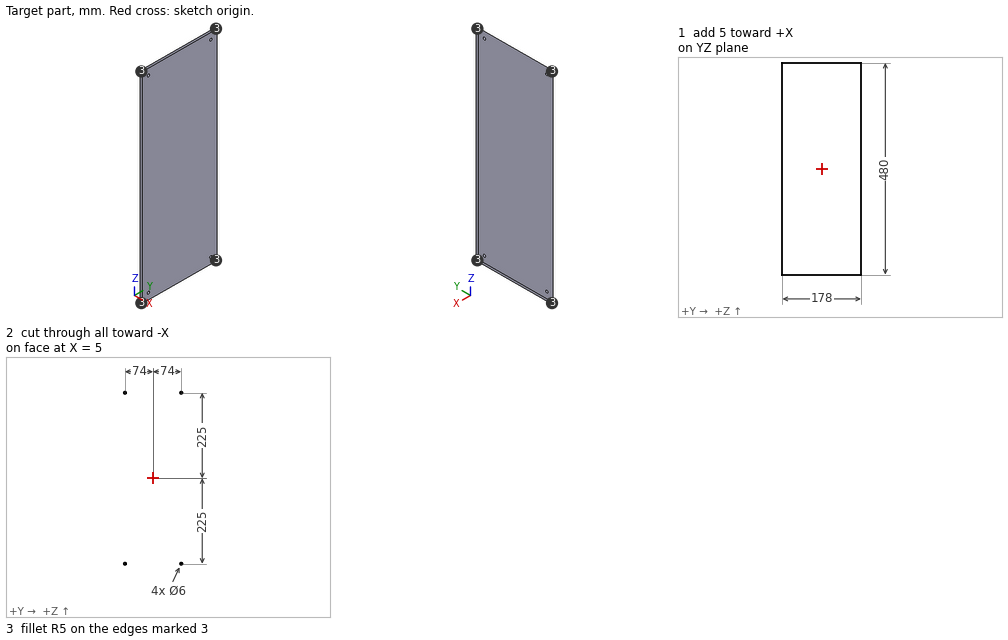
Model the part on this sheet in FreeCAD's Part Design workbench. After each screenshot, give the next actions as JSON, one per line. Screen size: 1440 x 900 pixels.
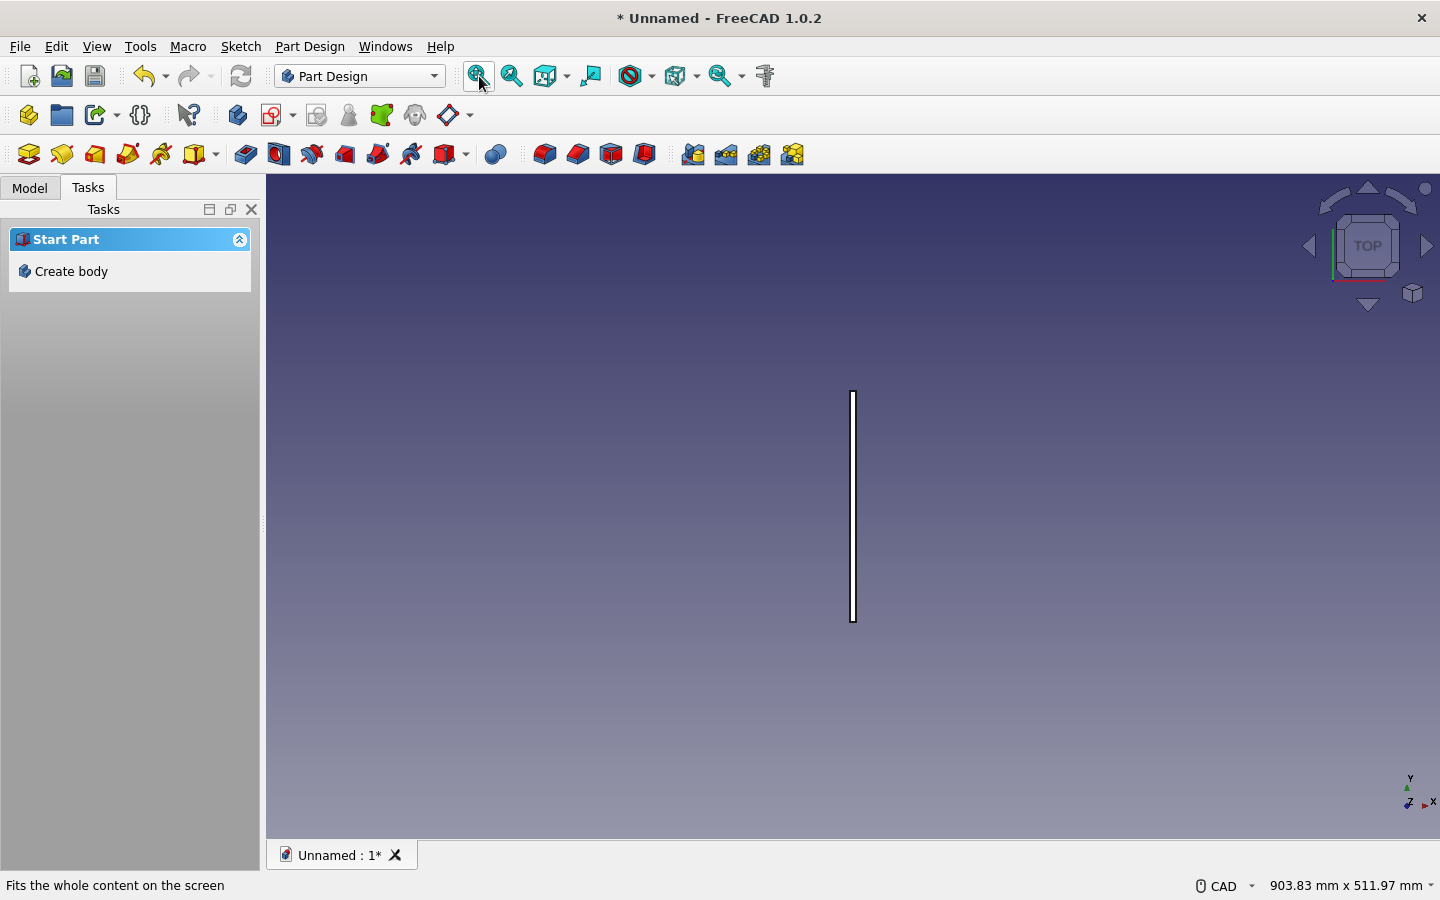
{"action": "left_click", "coordinate": [479, 76]}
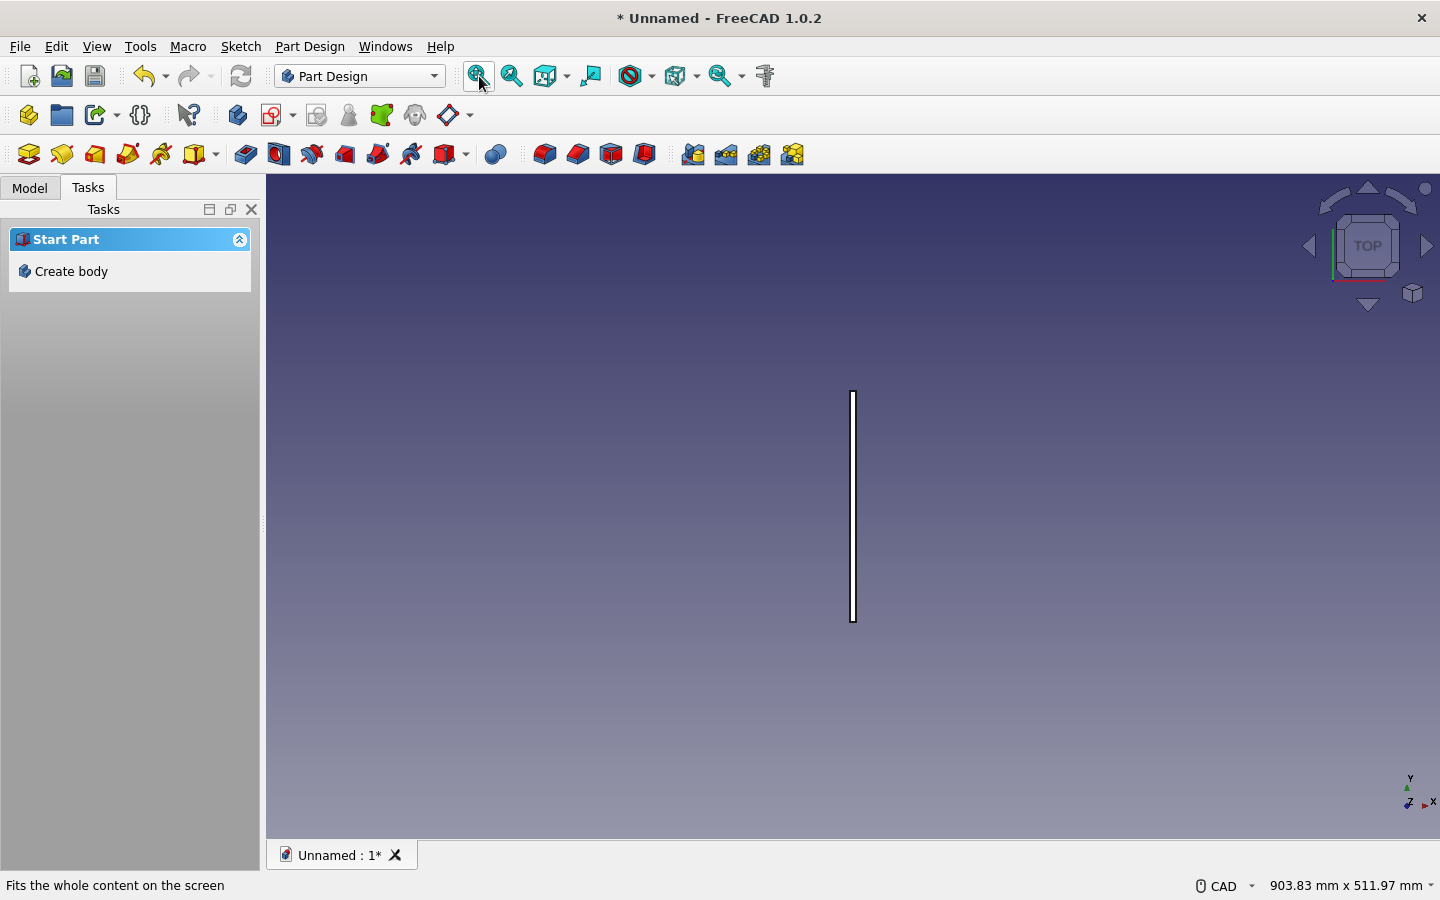
{"action": "scroll", "coordinate": [853, 390], "scroll_direction": "up", "scroll_amount": 10}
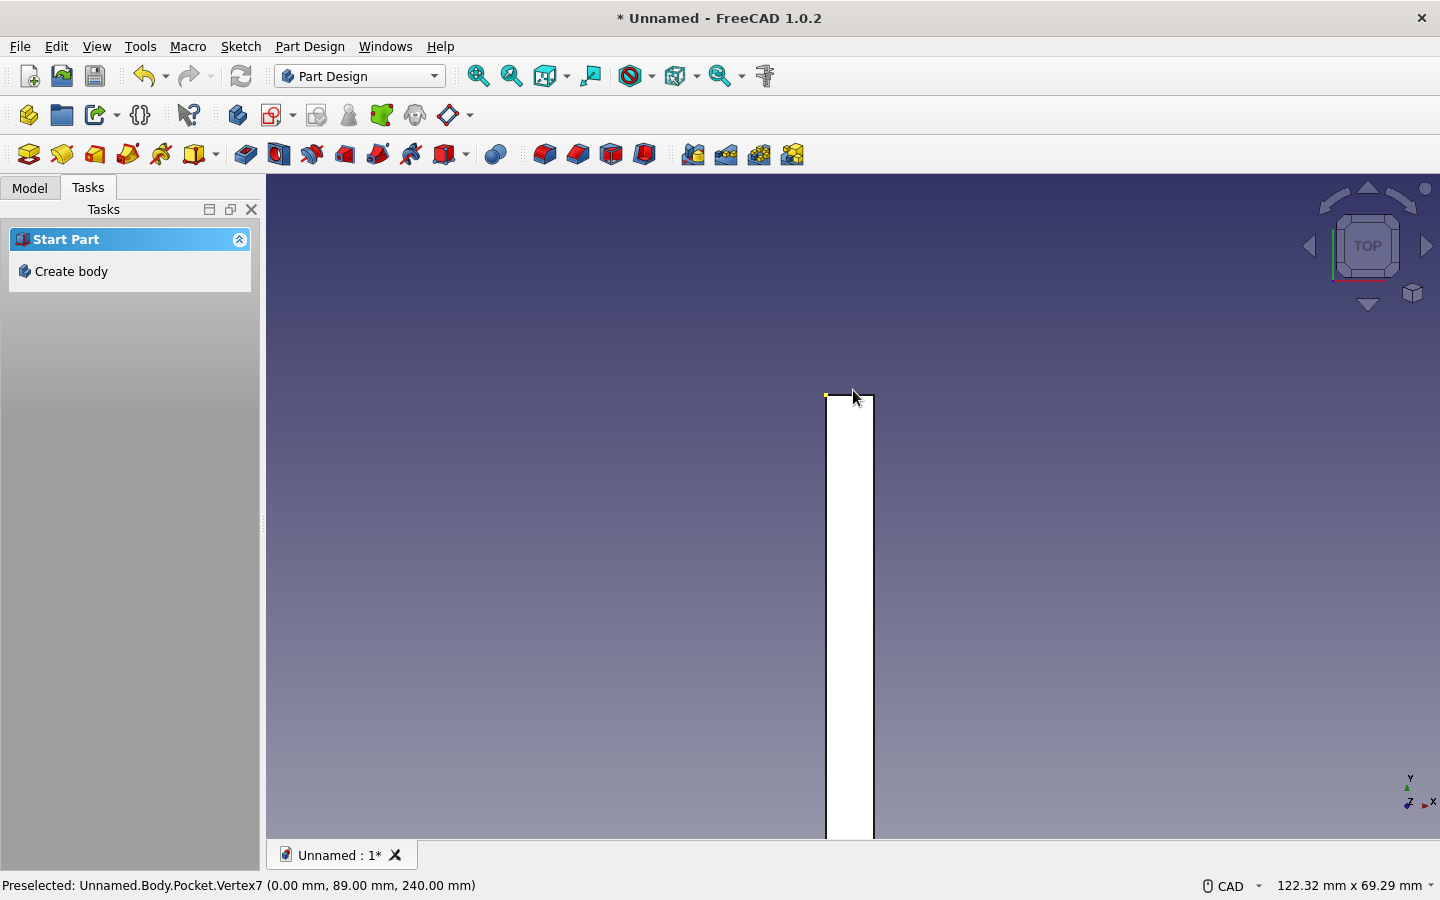
{"action": "left_click", "coordinate": [850, 394]}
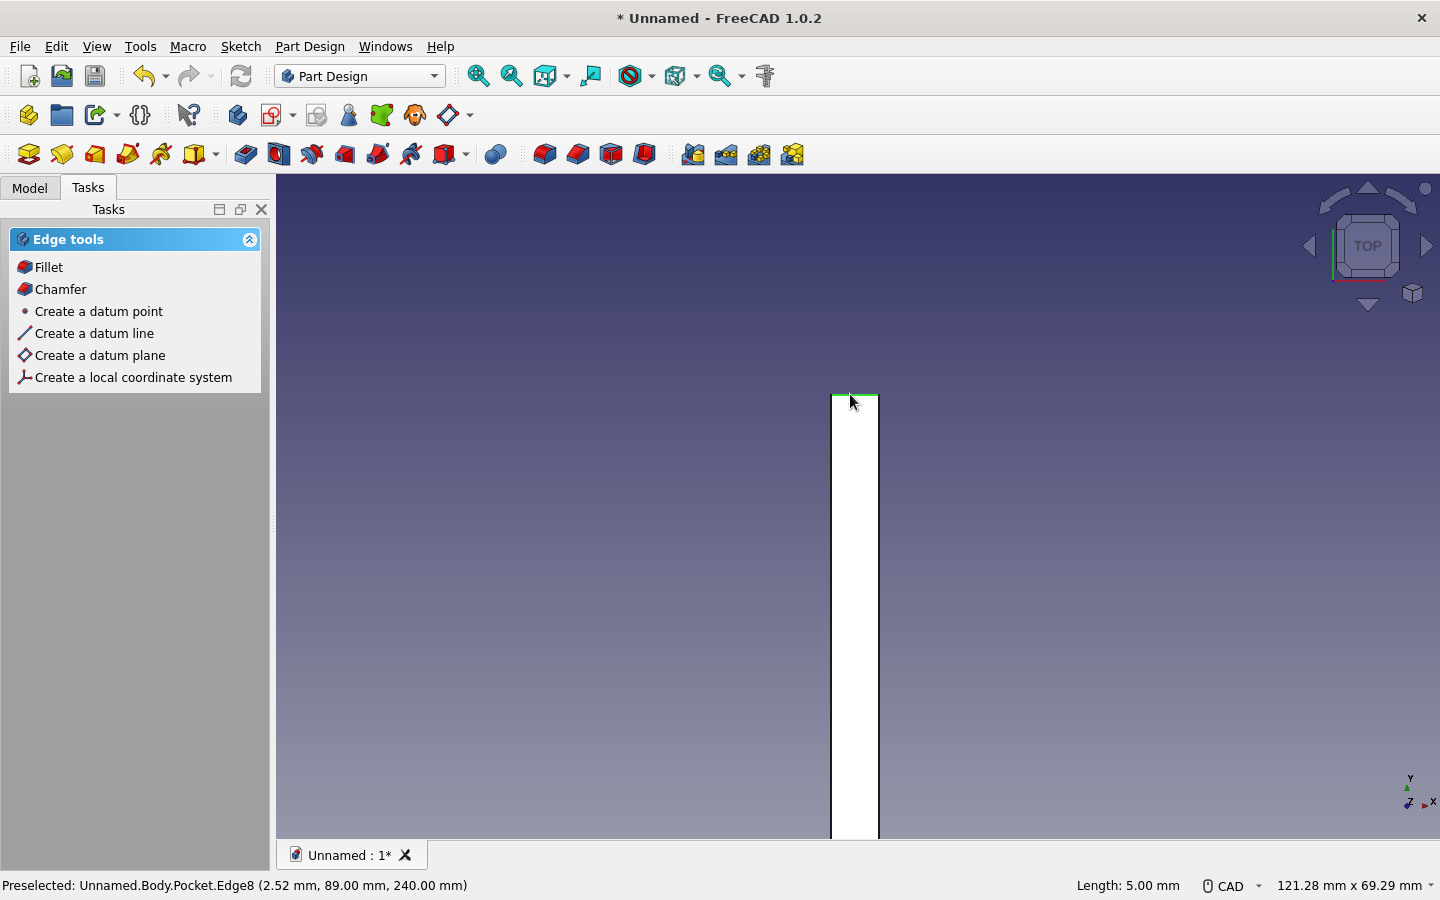
{"action": "left_click", "coordinate": [479, 76]}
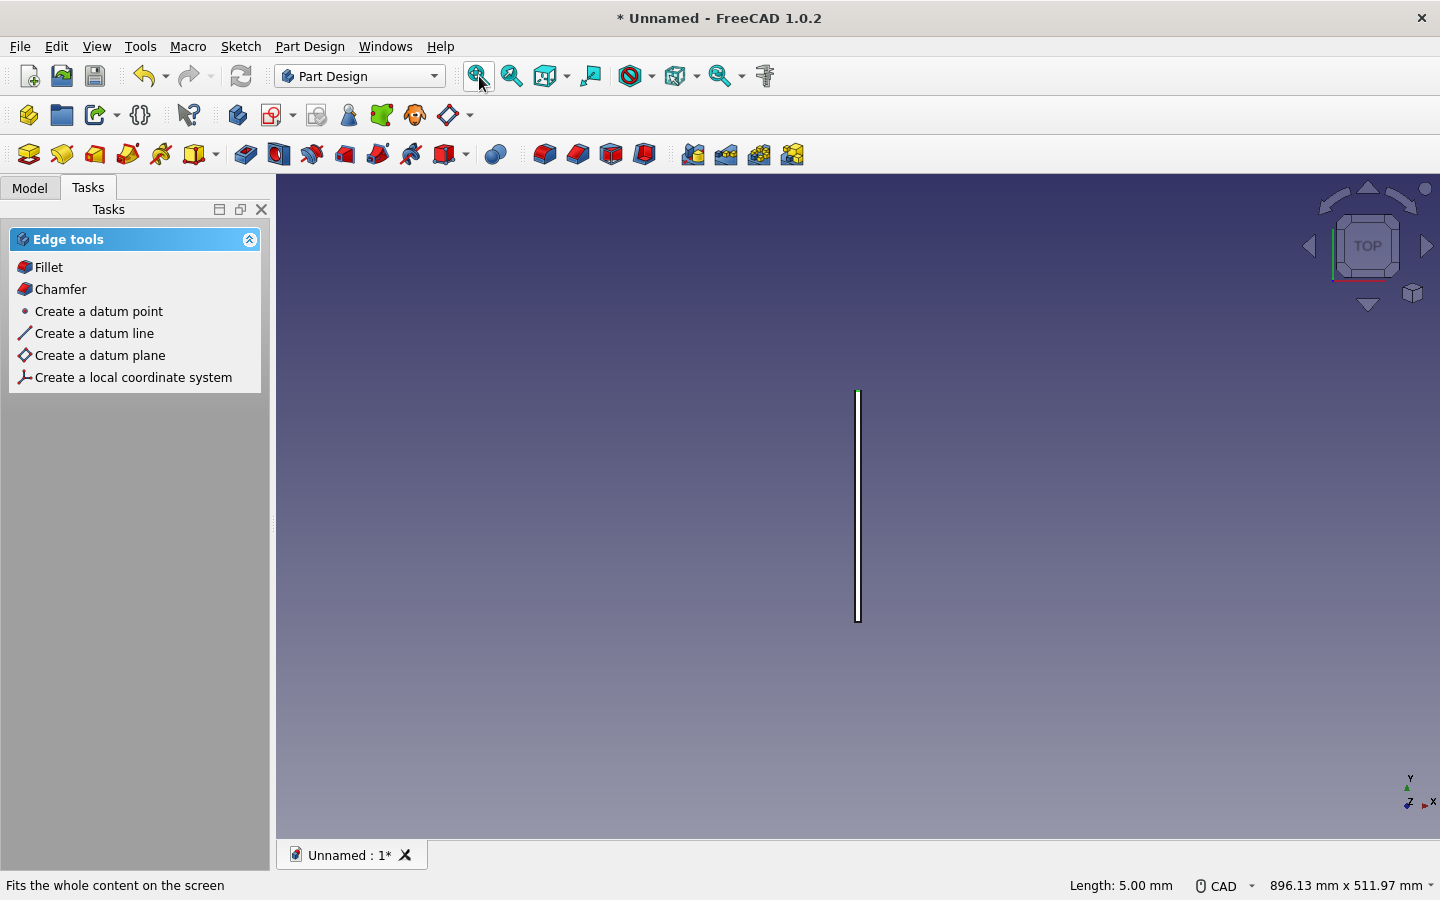
{"action": "key", "text": "1"}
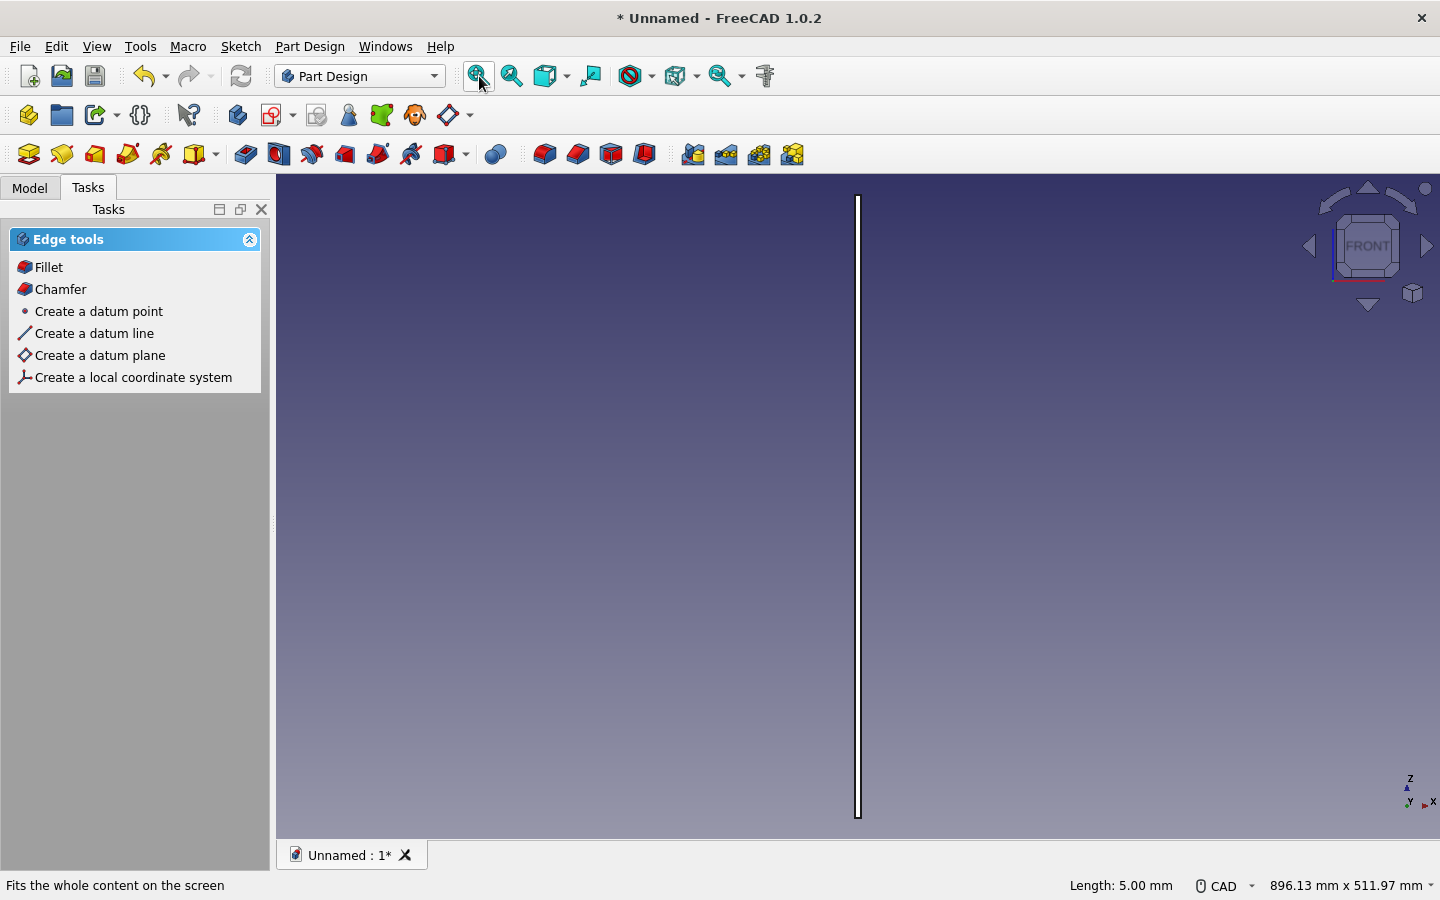
{"action": "key", "text": "3"}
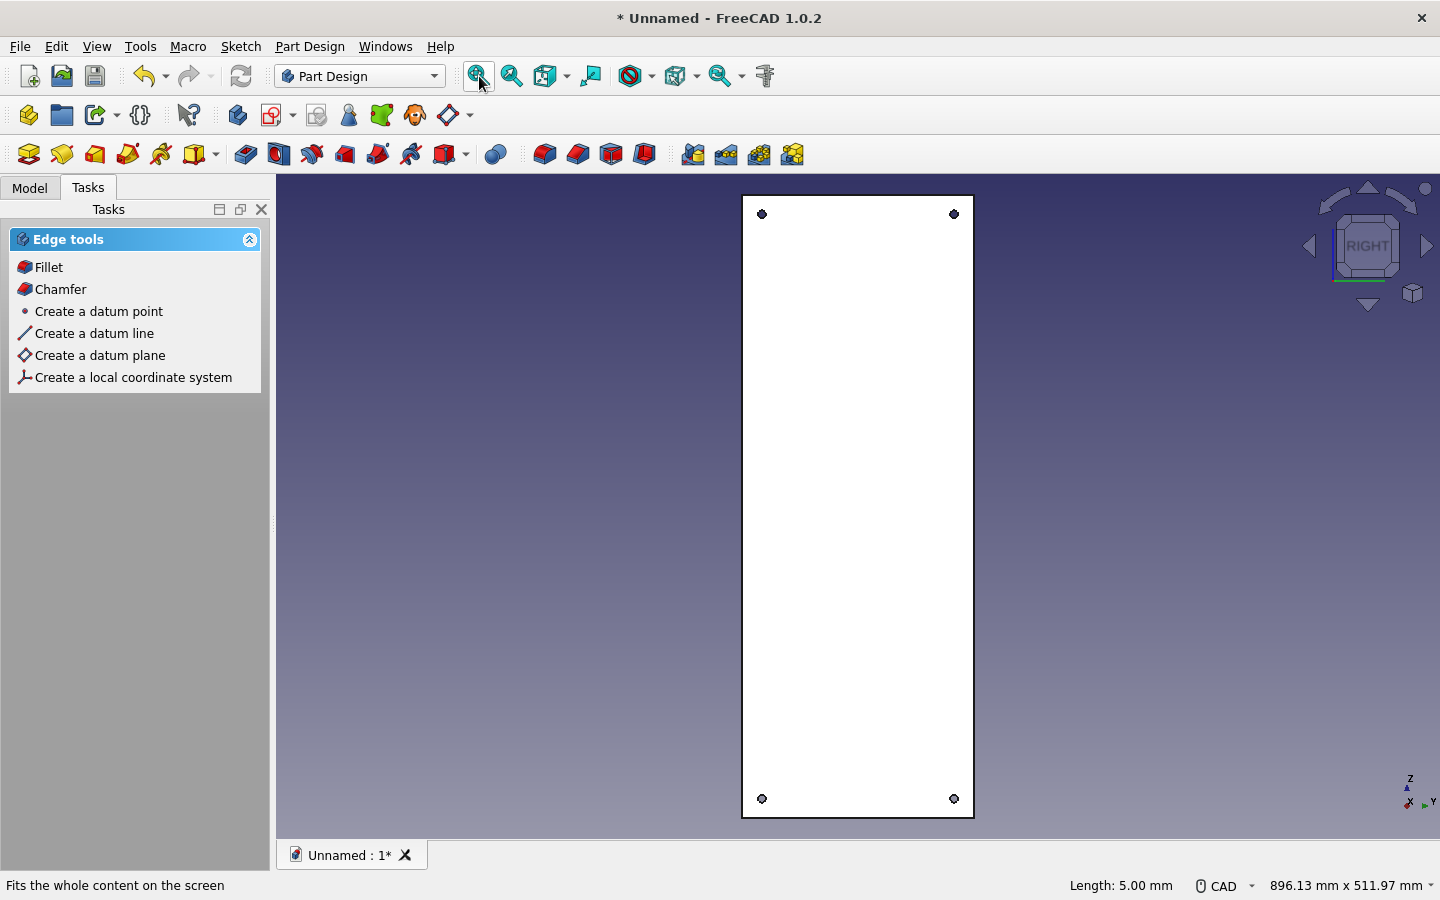
{"action": "key", "text": "5"}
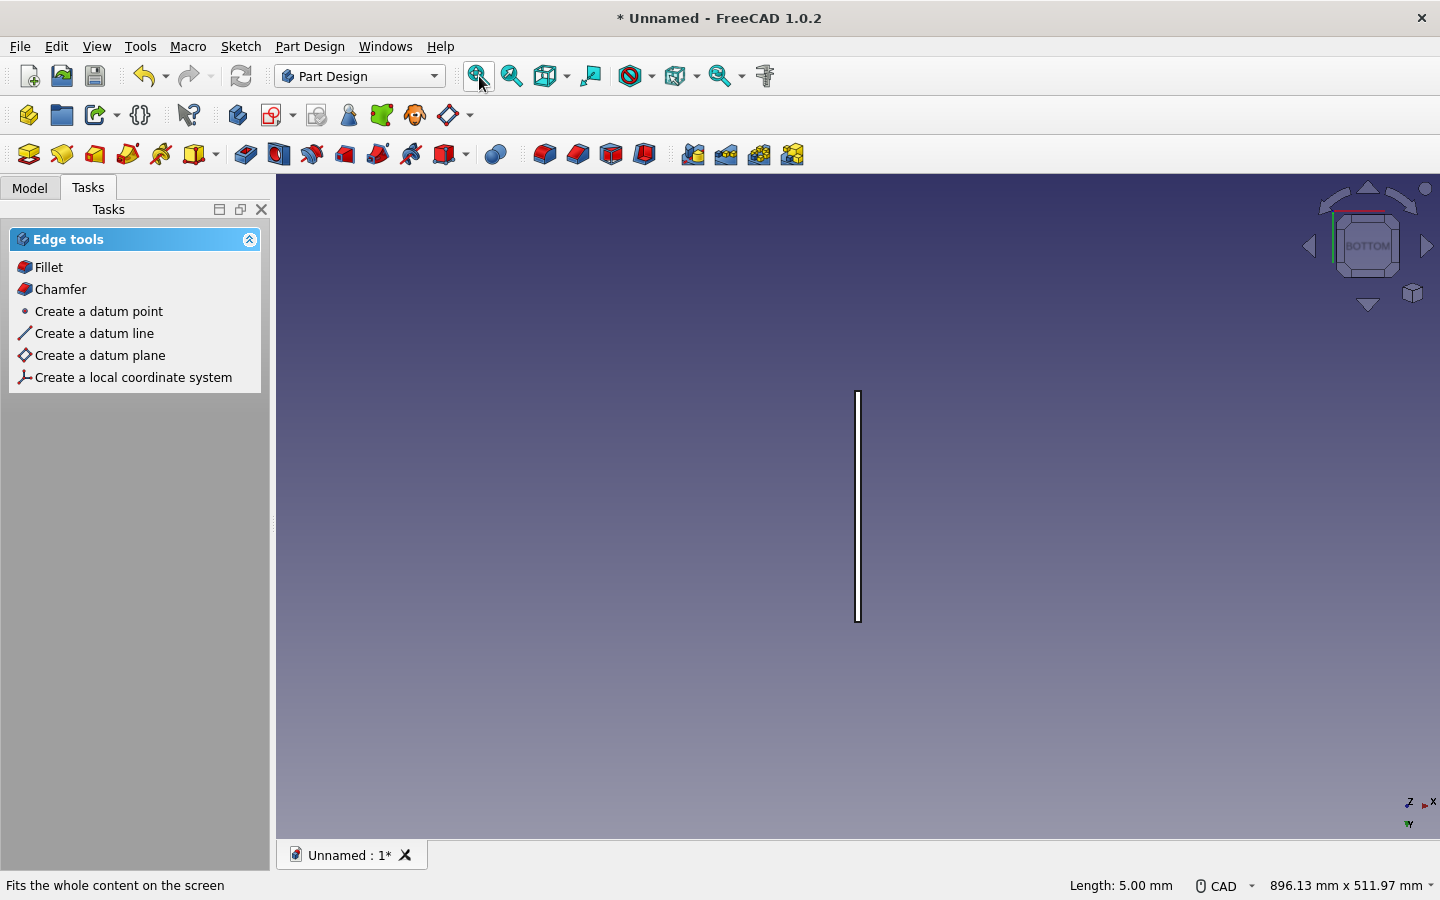
{"action": "left_click", "coordinate": [479, 76]}